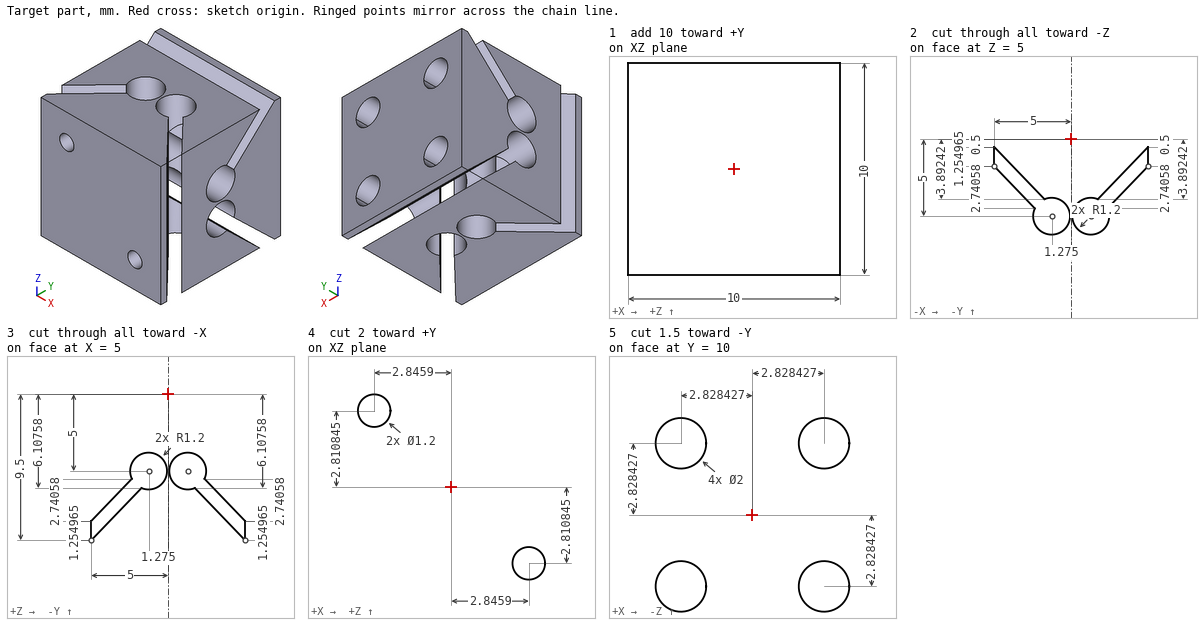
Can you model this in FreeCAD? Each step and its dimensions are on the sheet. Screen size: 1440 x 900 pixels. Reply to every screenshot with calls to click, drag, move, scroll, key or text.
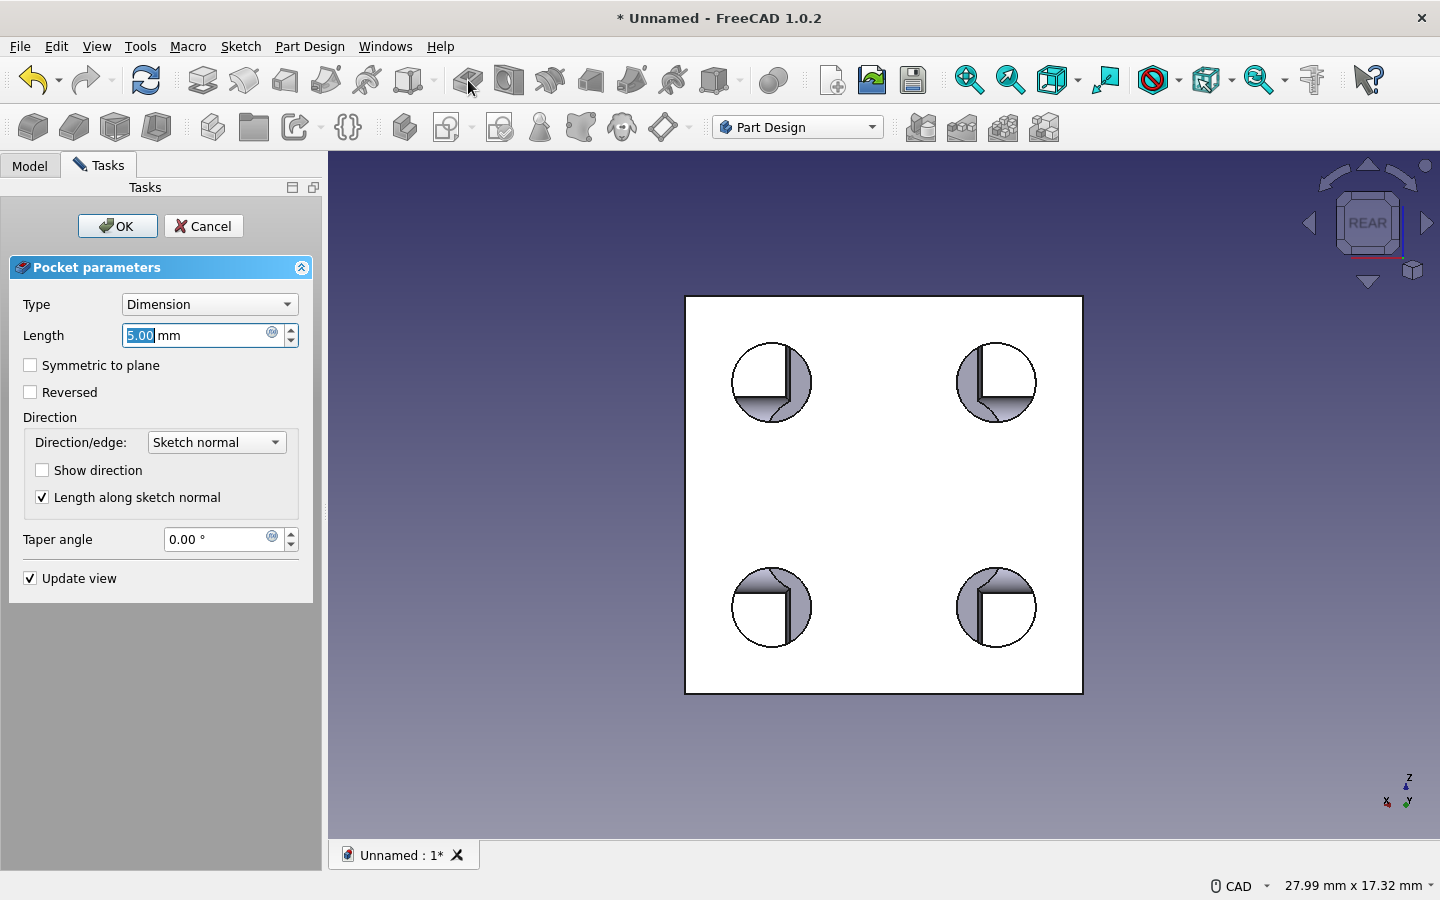
text(1.5)
key(Tab)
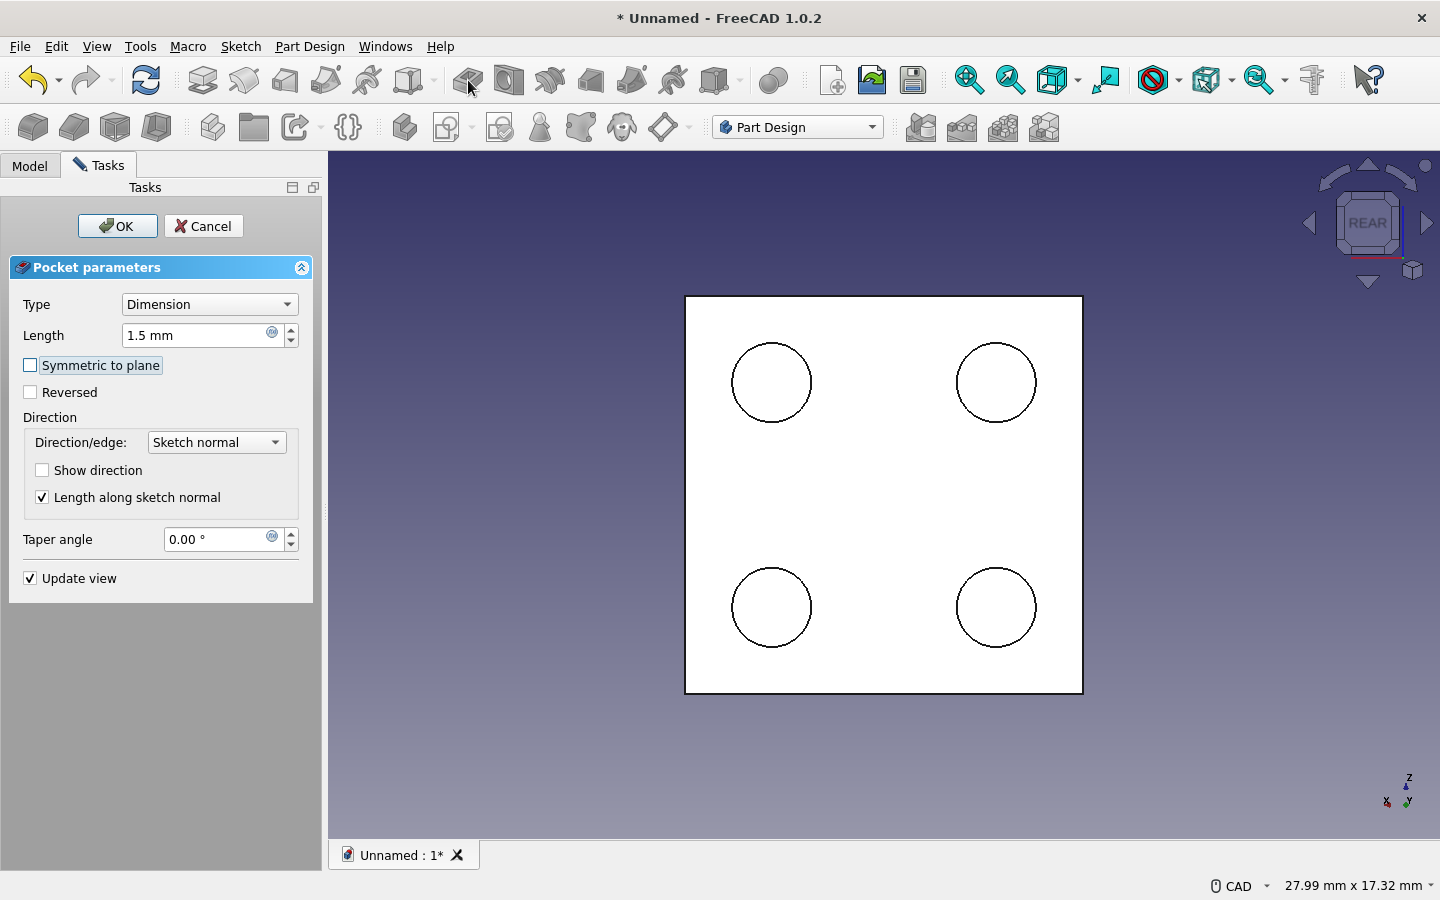
click(118, 226)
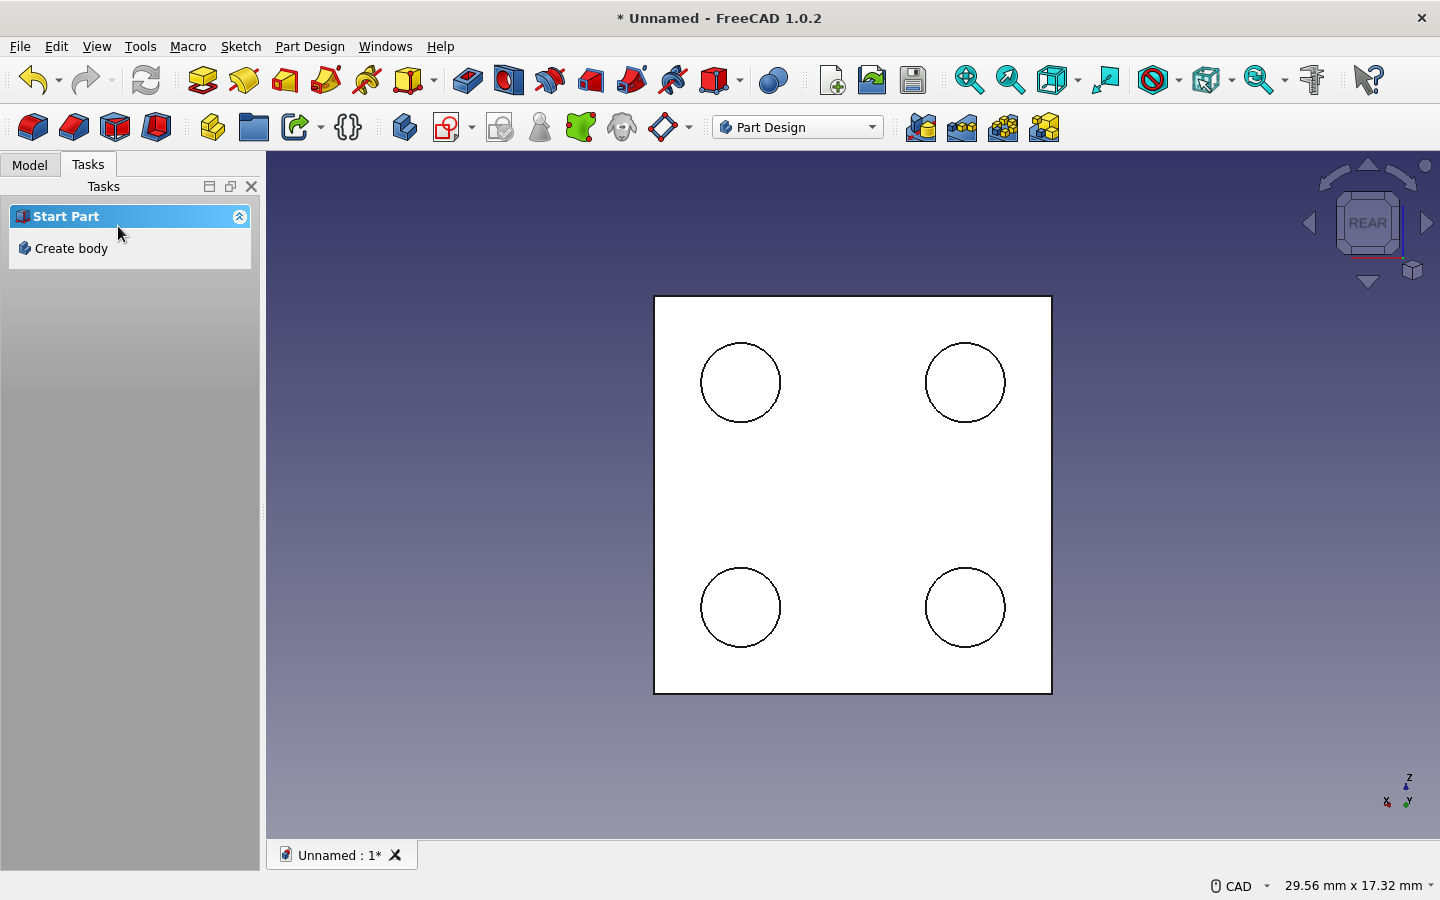
key(0)